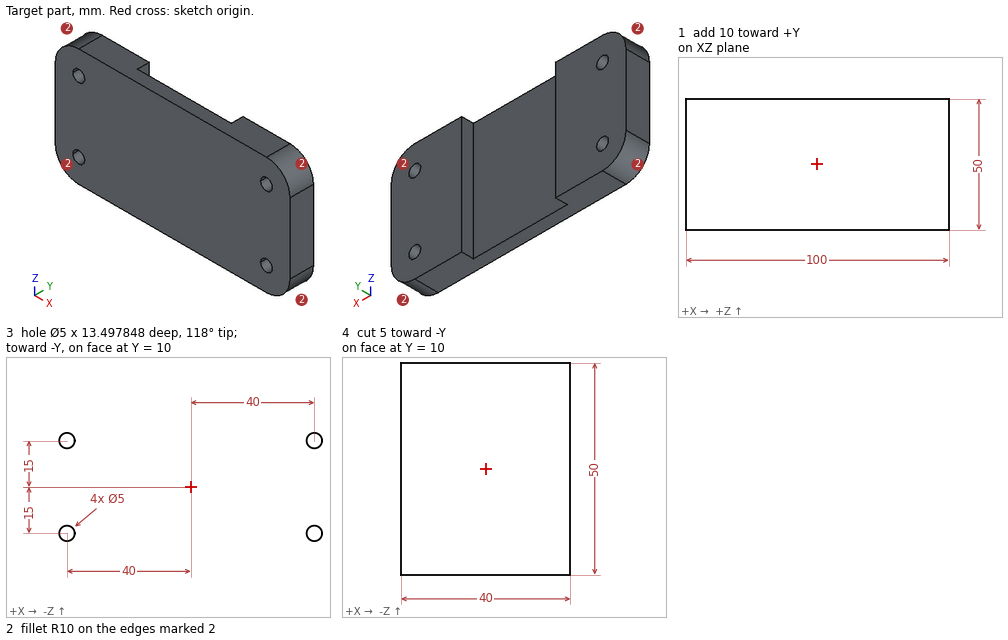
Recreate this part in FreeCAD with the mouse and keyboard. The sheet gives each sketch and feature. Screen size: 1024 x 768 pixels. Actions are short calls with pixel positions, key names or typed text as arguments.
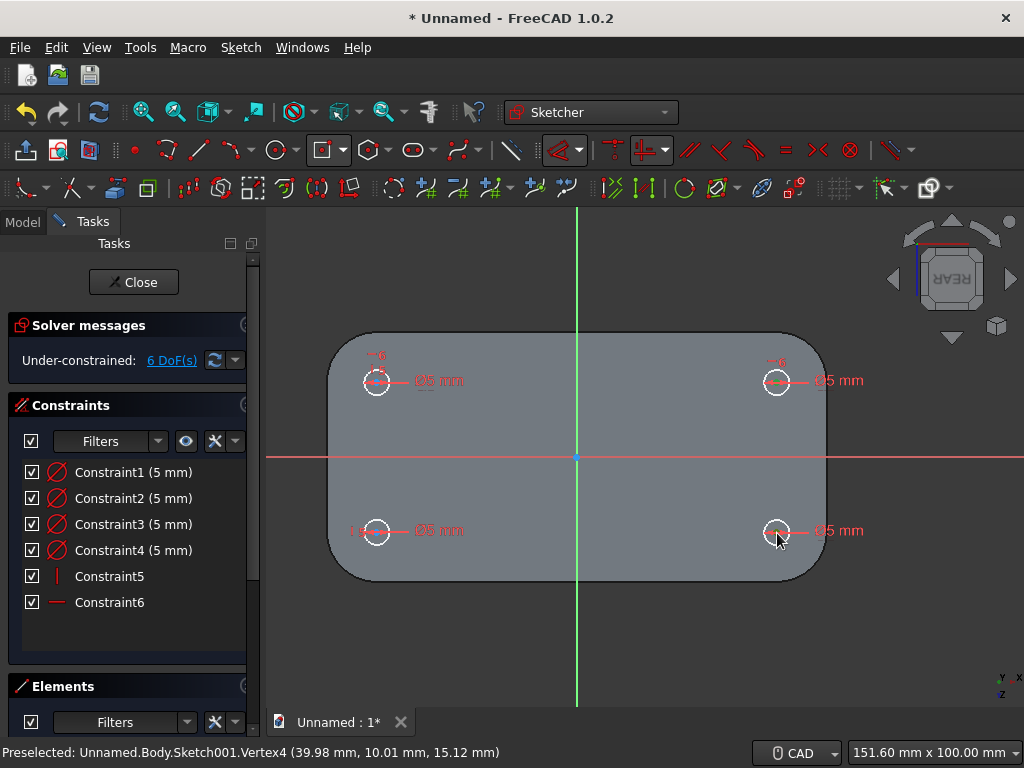
key(v)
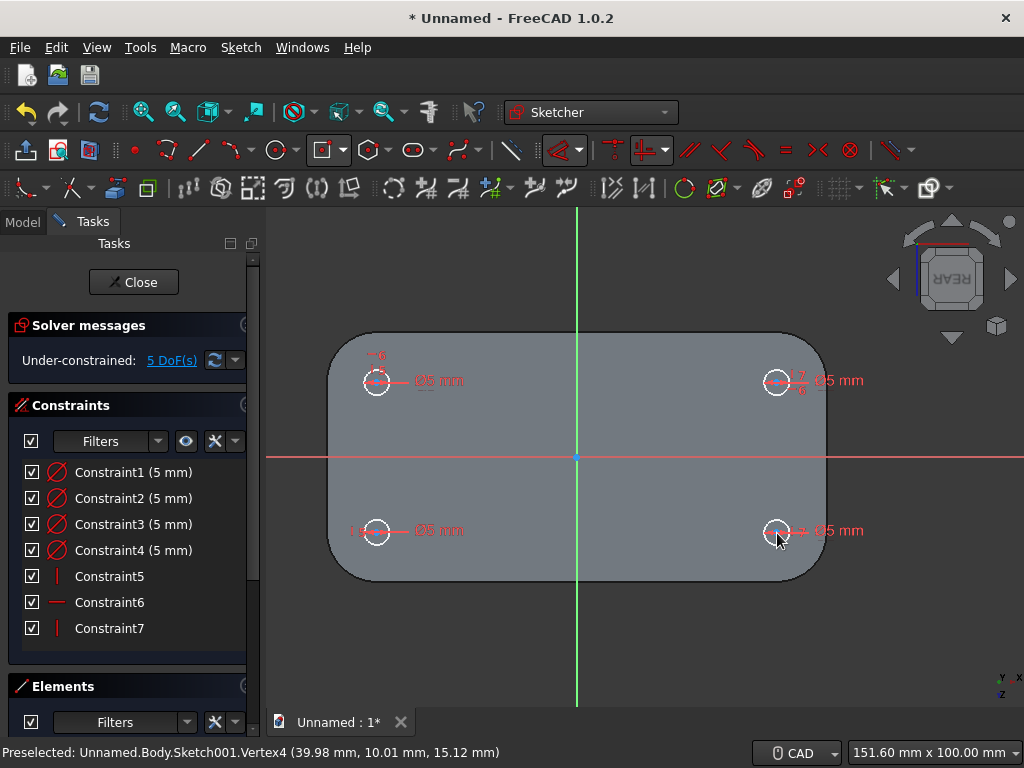
click(377, 532)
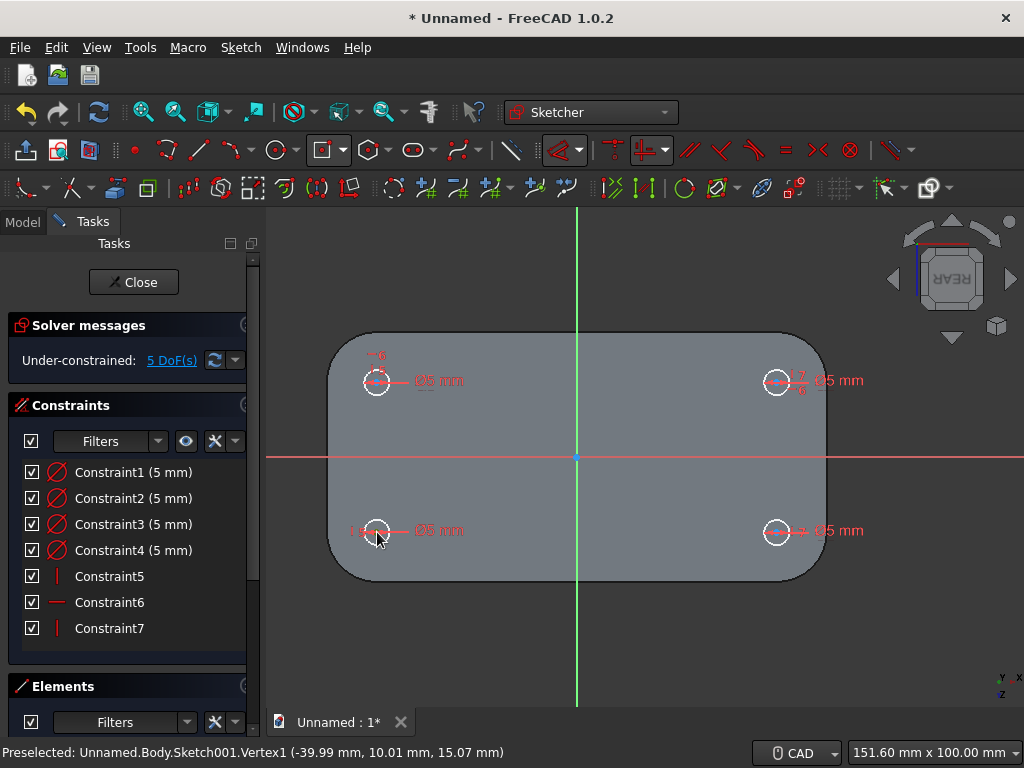
click(777, 533)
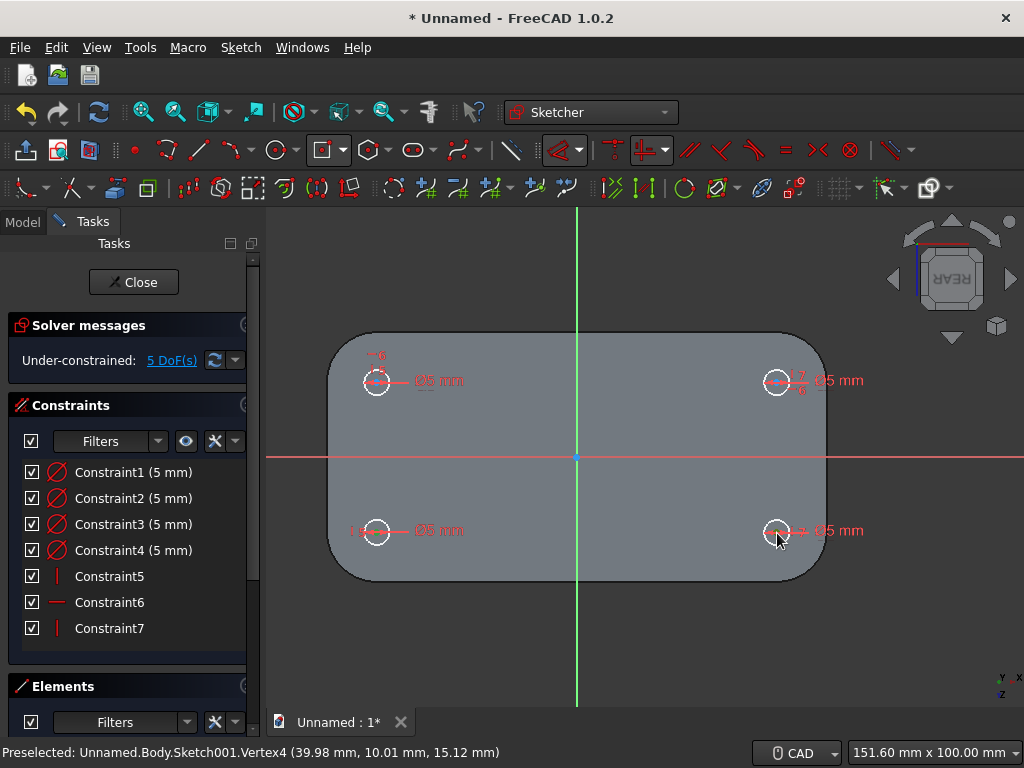
click(668, 150)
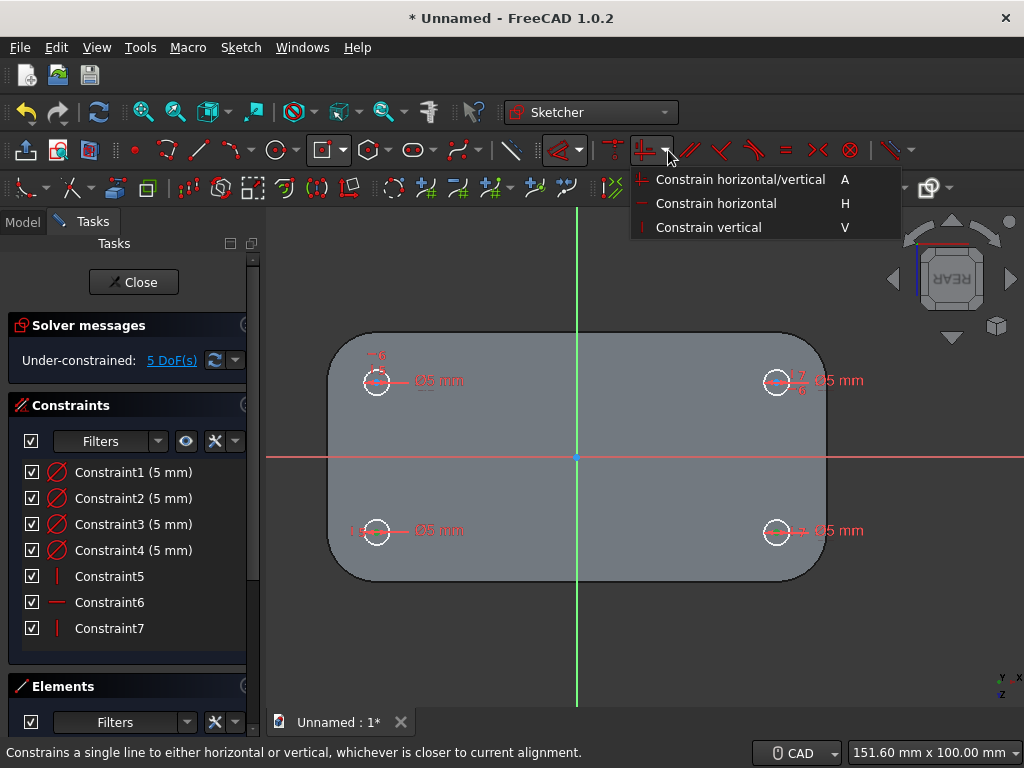
click(766, 203)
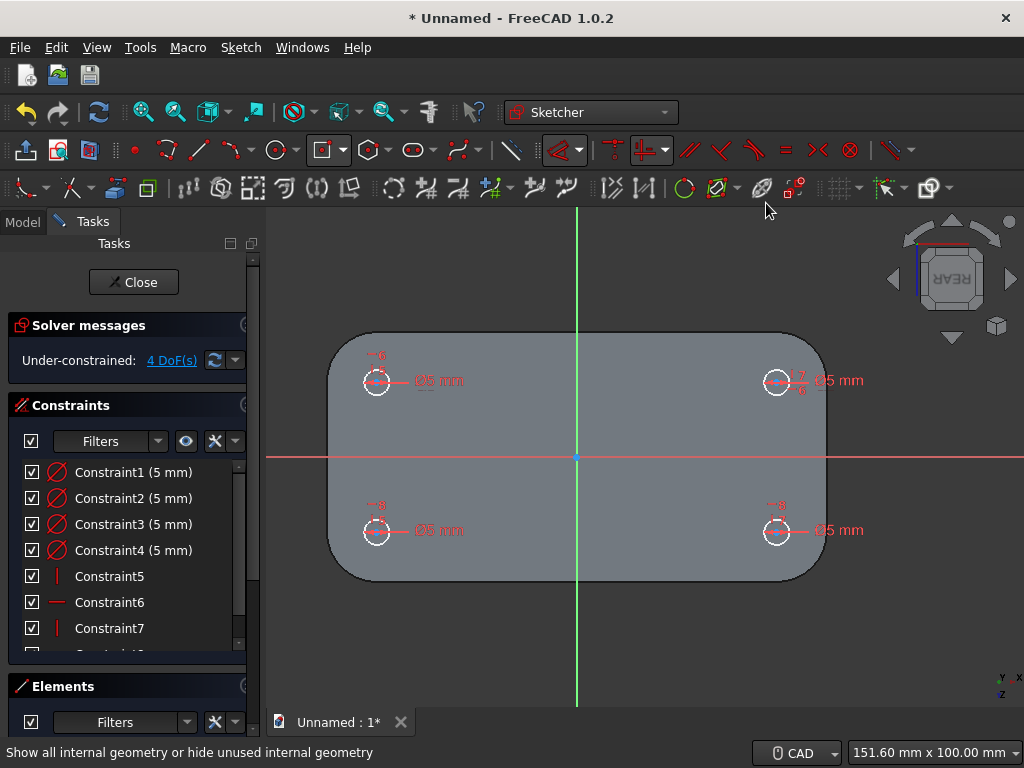
click(558, 150)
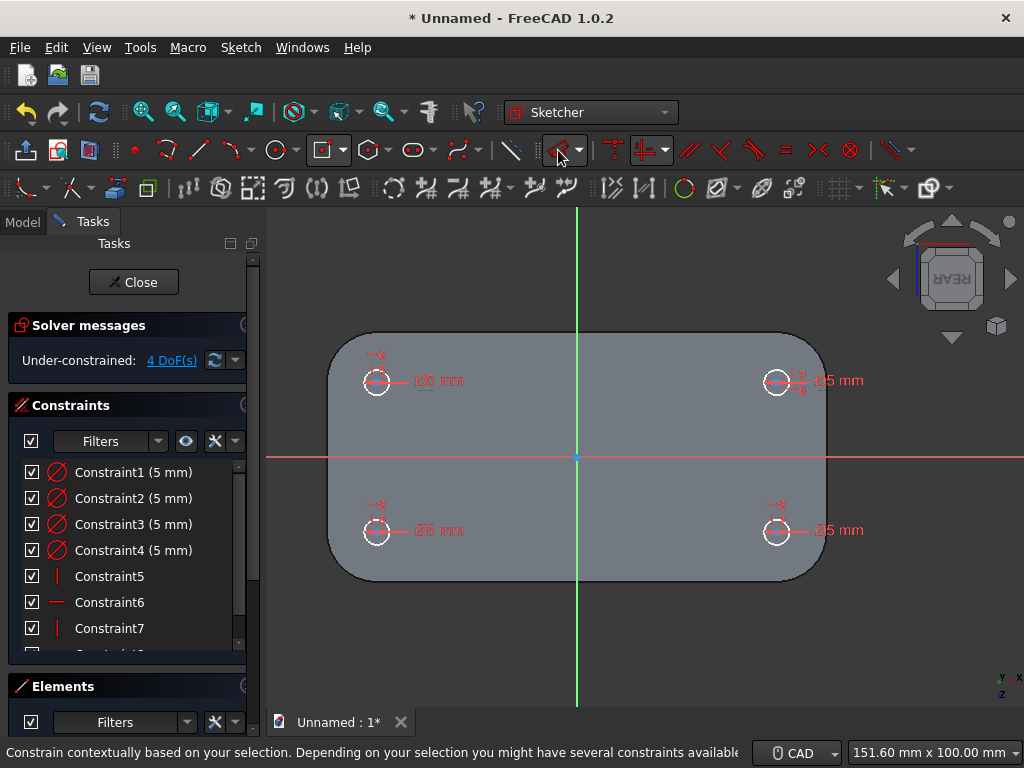
click(377, 532)
click(477, 566)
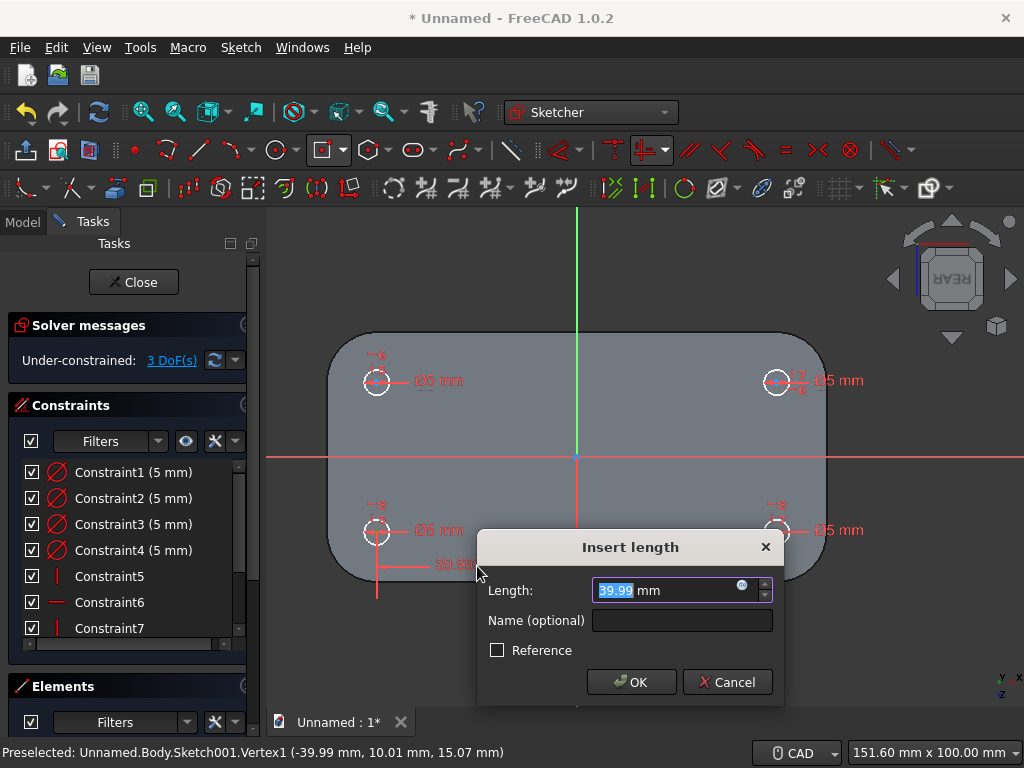
text(40)
key(Return)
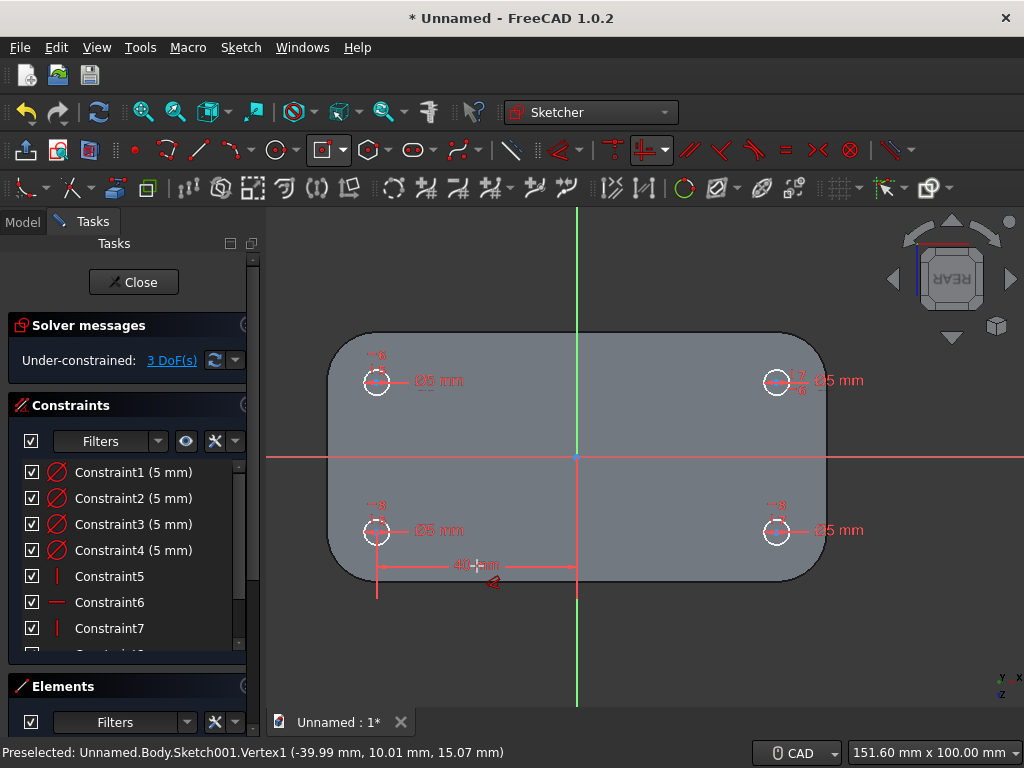
click(377, 532)
click(343, 495)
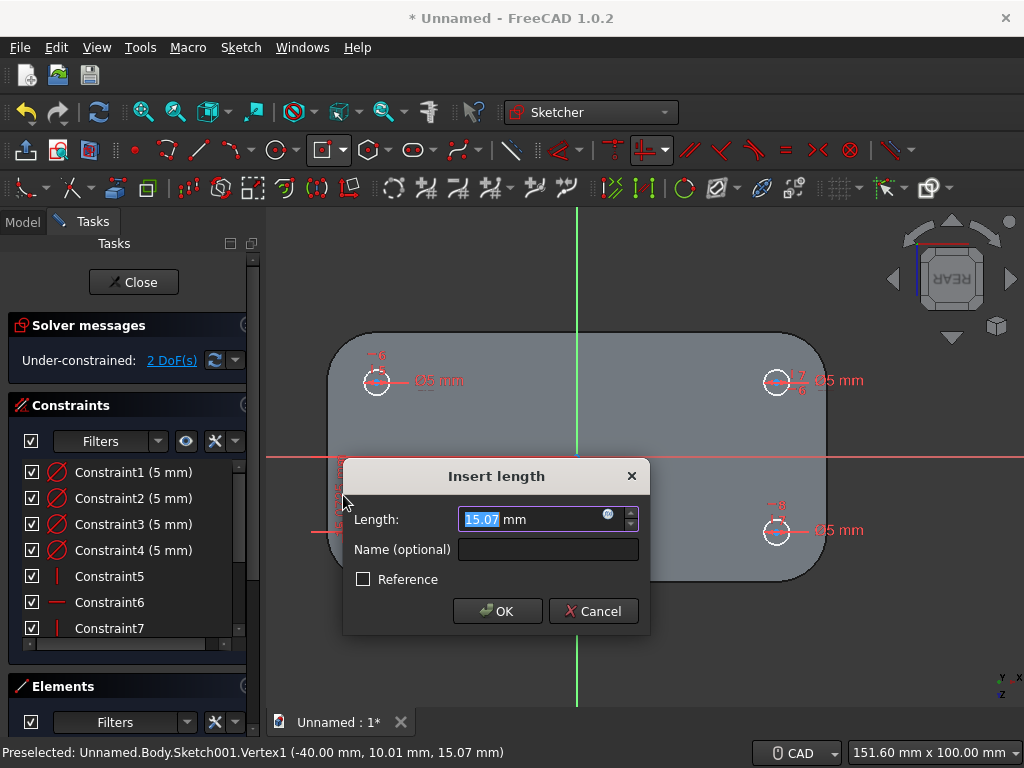
text(15)
key(Return)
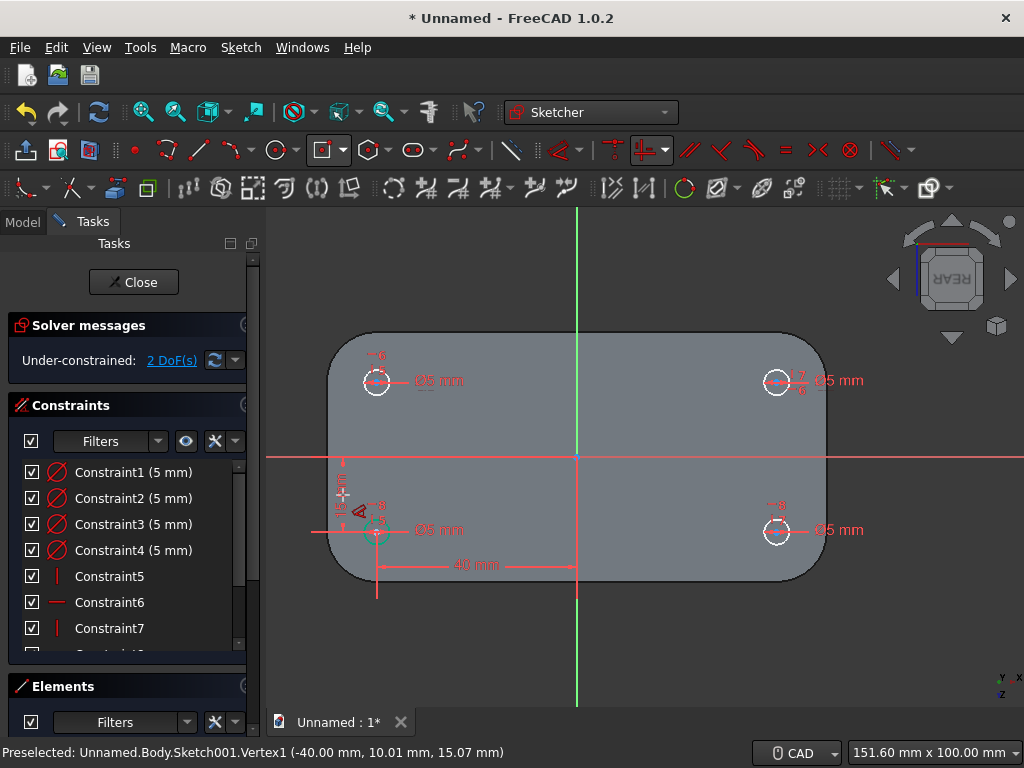
click(377, 383)
click(343, 420)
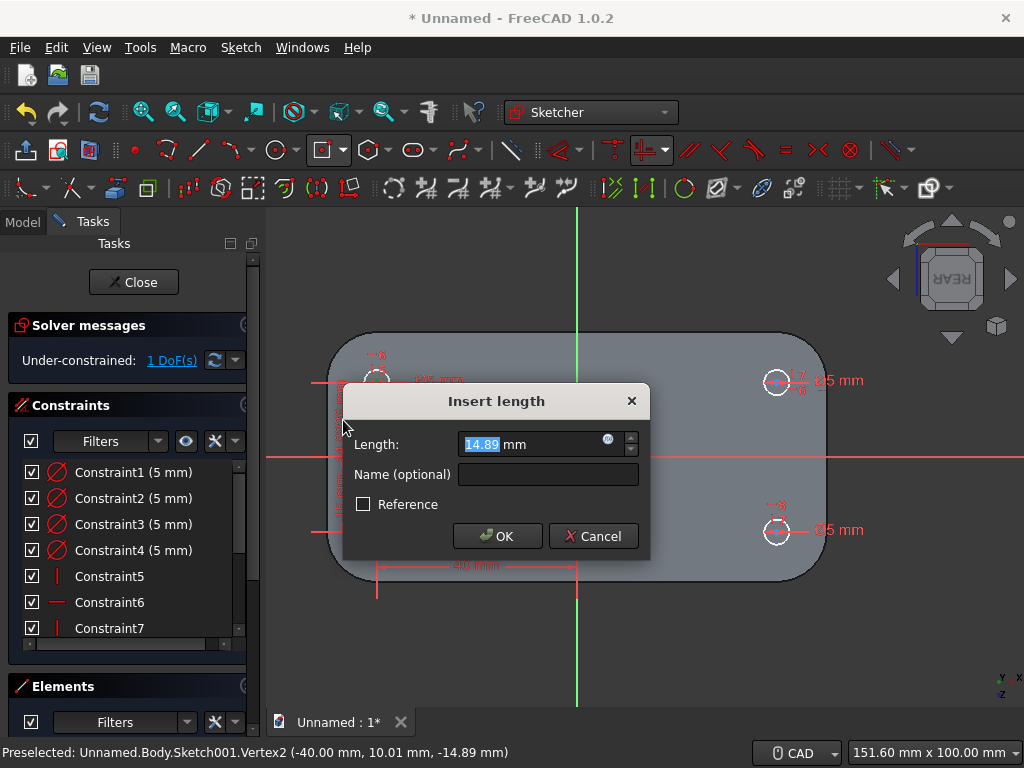
text(15)
key(Return)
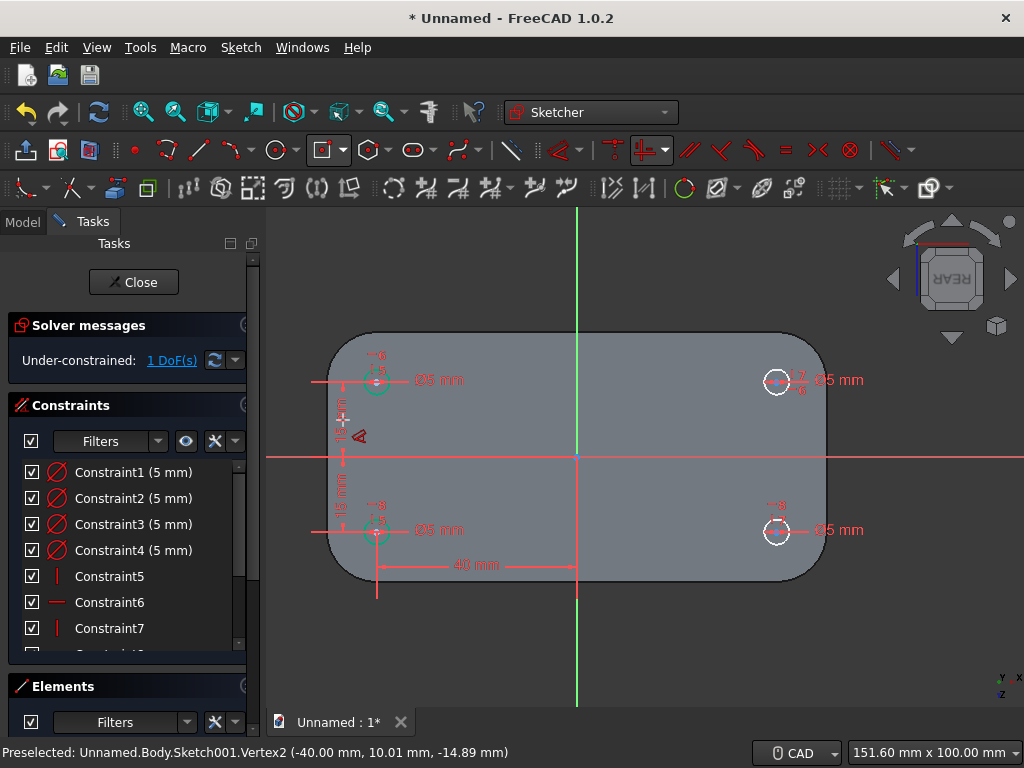
click(777, 382)
click(677, 348)